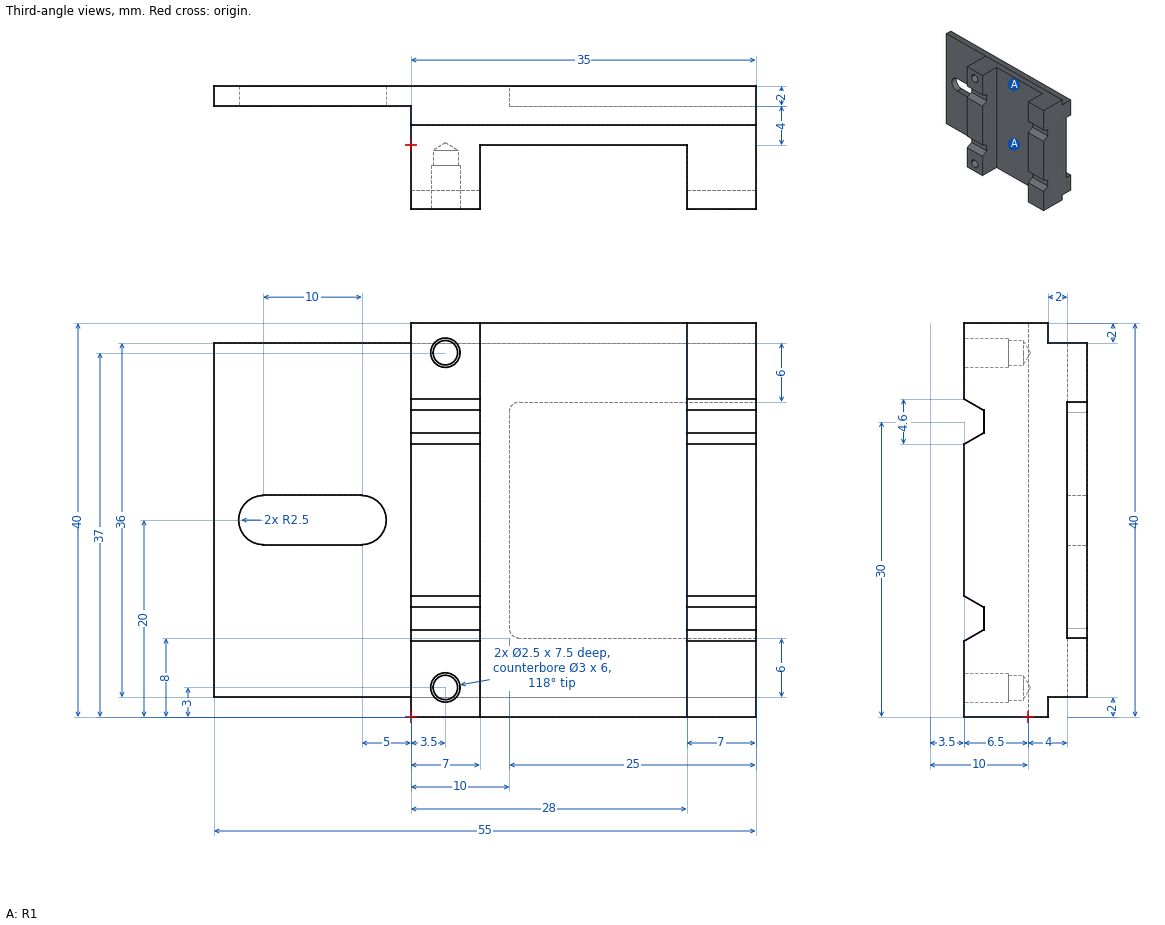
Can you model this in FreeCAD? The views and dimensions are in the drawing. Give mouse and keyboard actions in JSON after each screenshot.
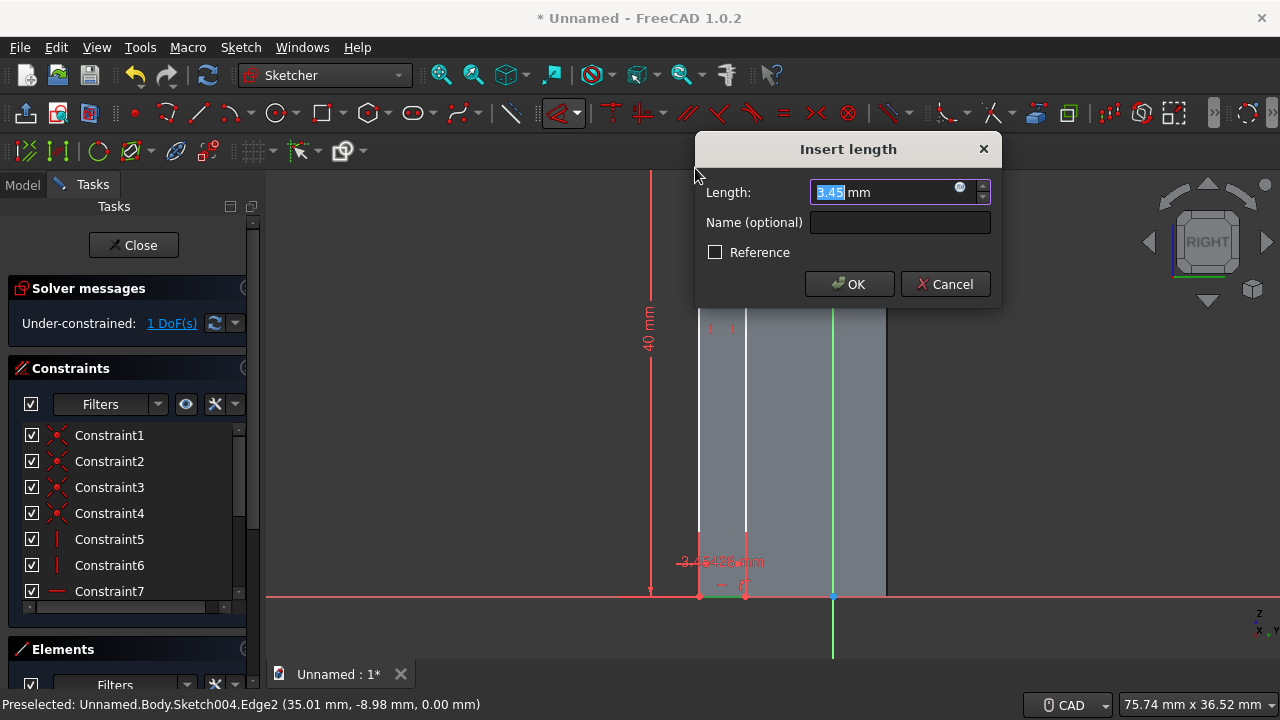
{"action": "type", "text": "3.5"}
{"action": "key", "text": "Return"}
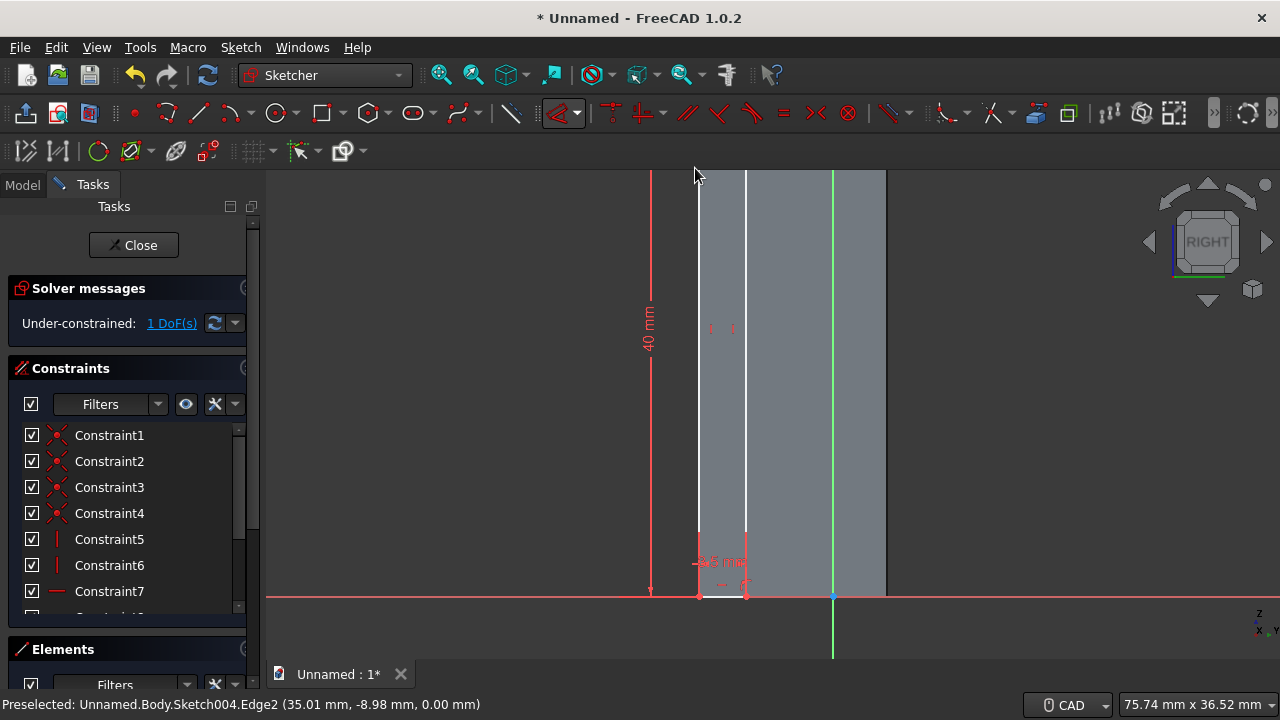
{"action": "scroll", "coordinate": [629, 519], "scroll_direction": "down", "scroll_amount": 3}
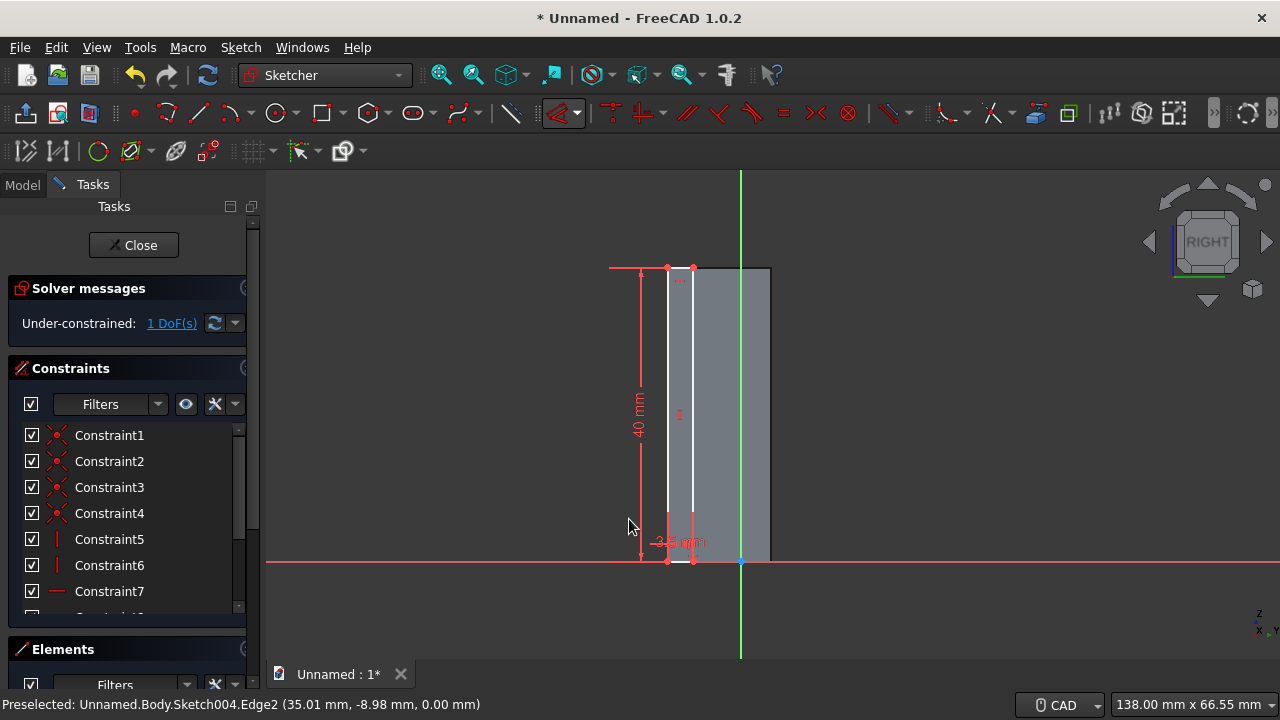
{"action": "left_click", "coordinate": [668, 268]}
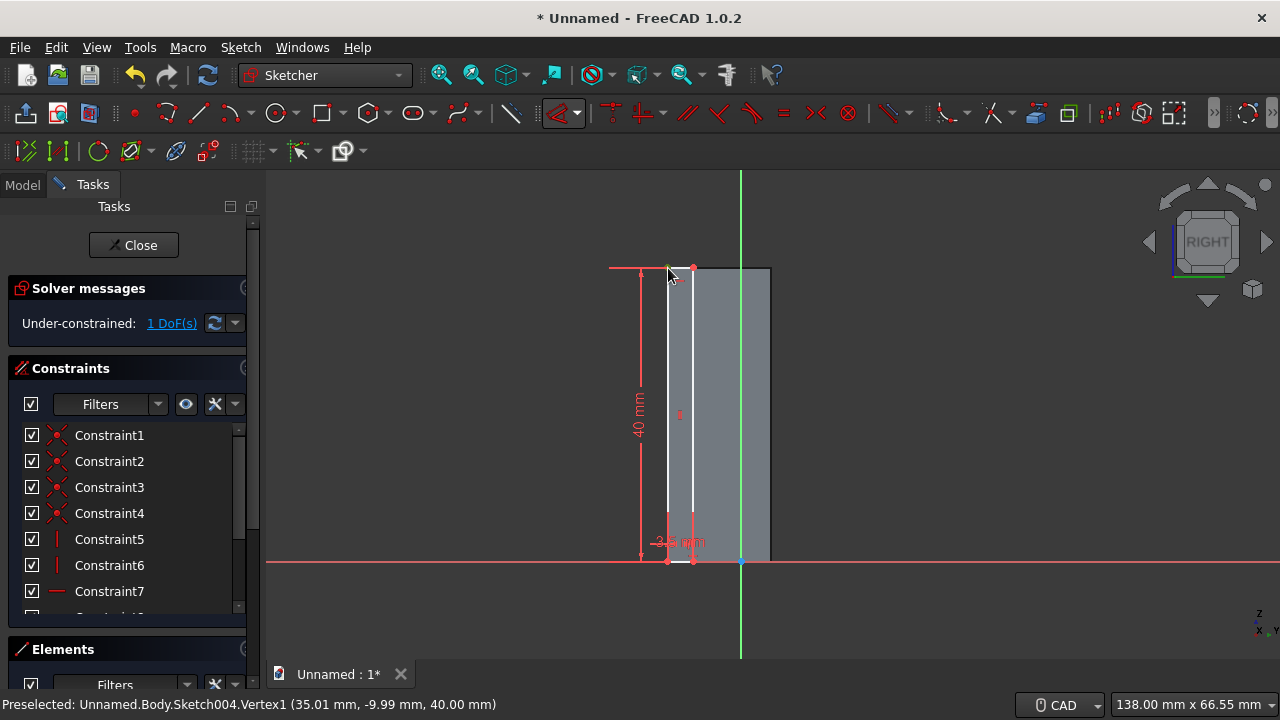
{"action": "left_click", "coordinate": [580, 114]}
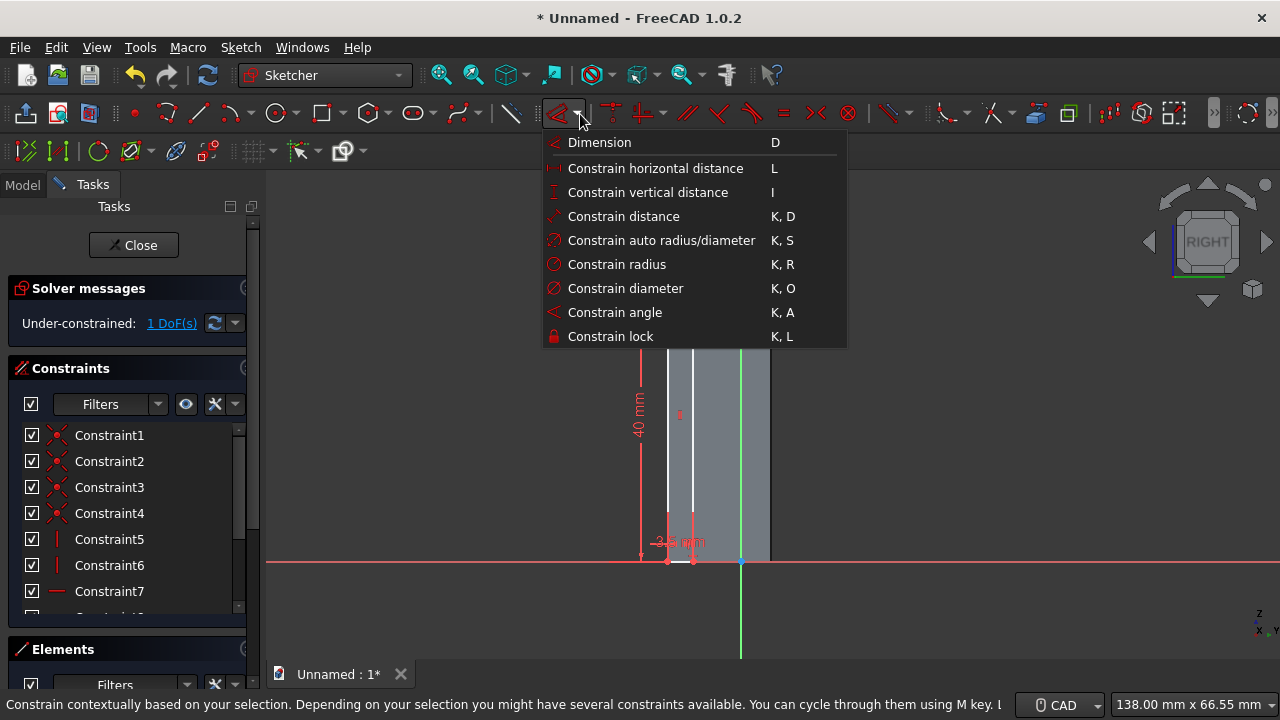
{"action": "left_click", "coordinate": [695, 168]}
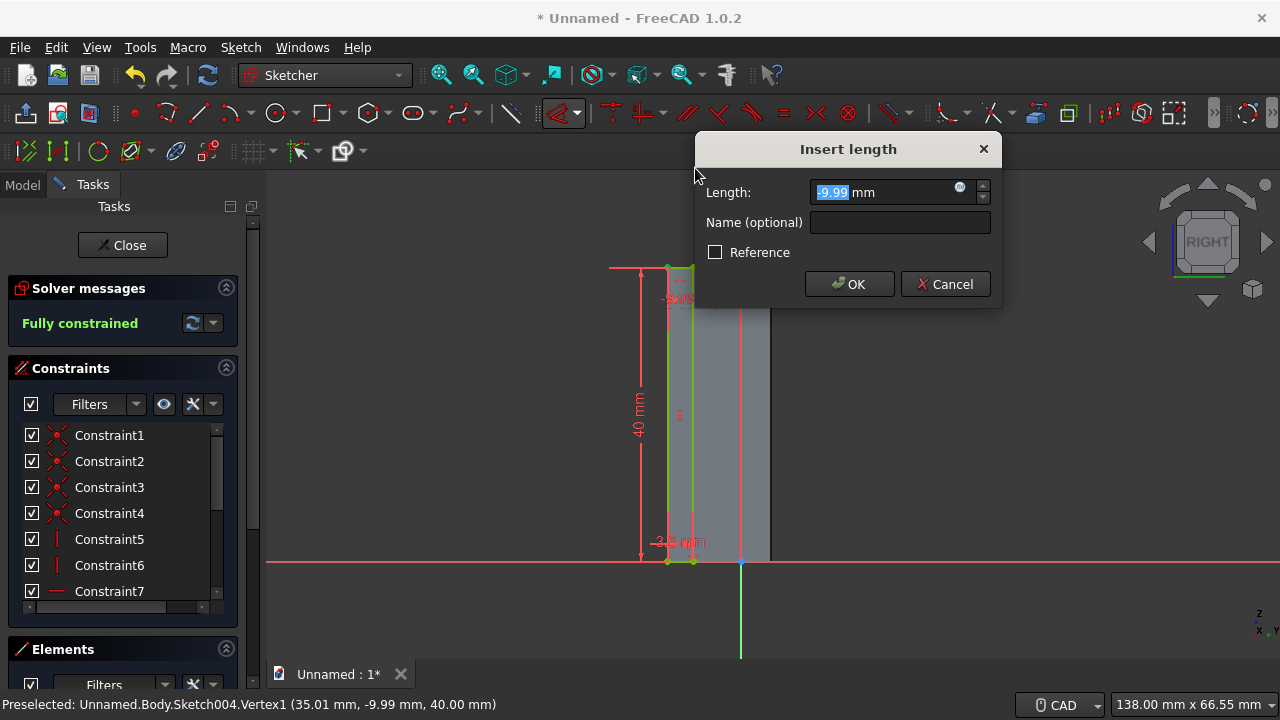
{"action": "type", "text": "-10"}
{"action": "key", "text": "Return"}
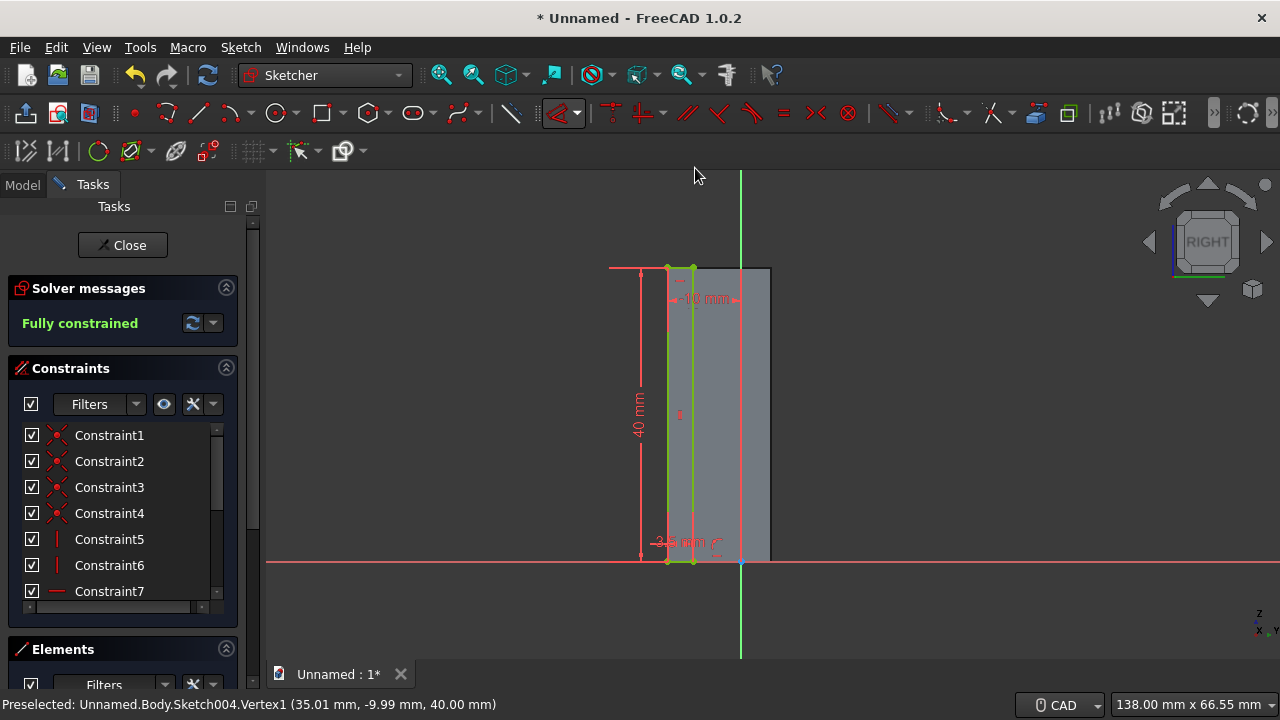
{"action": "left_click", "coordinate": [123, 245]}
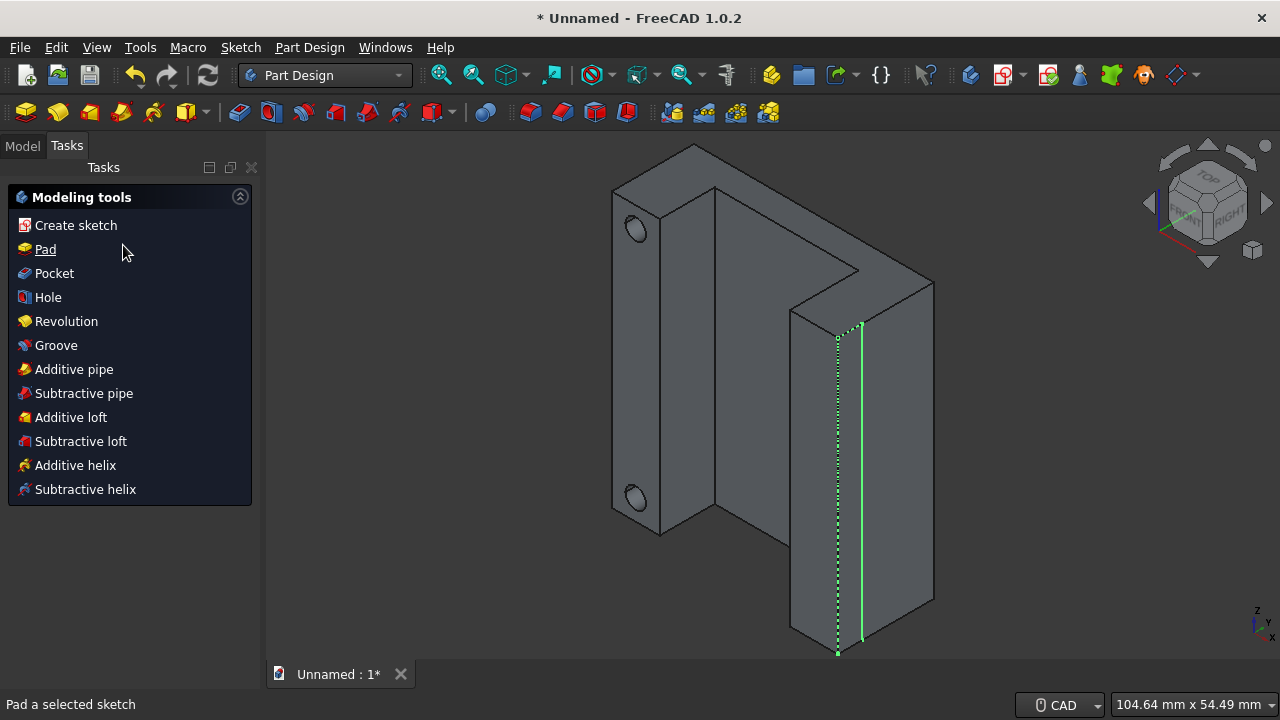
{"action": "left_click", "coordinate": [240, 112]}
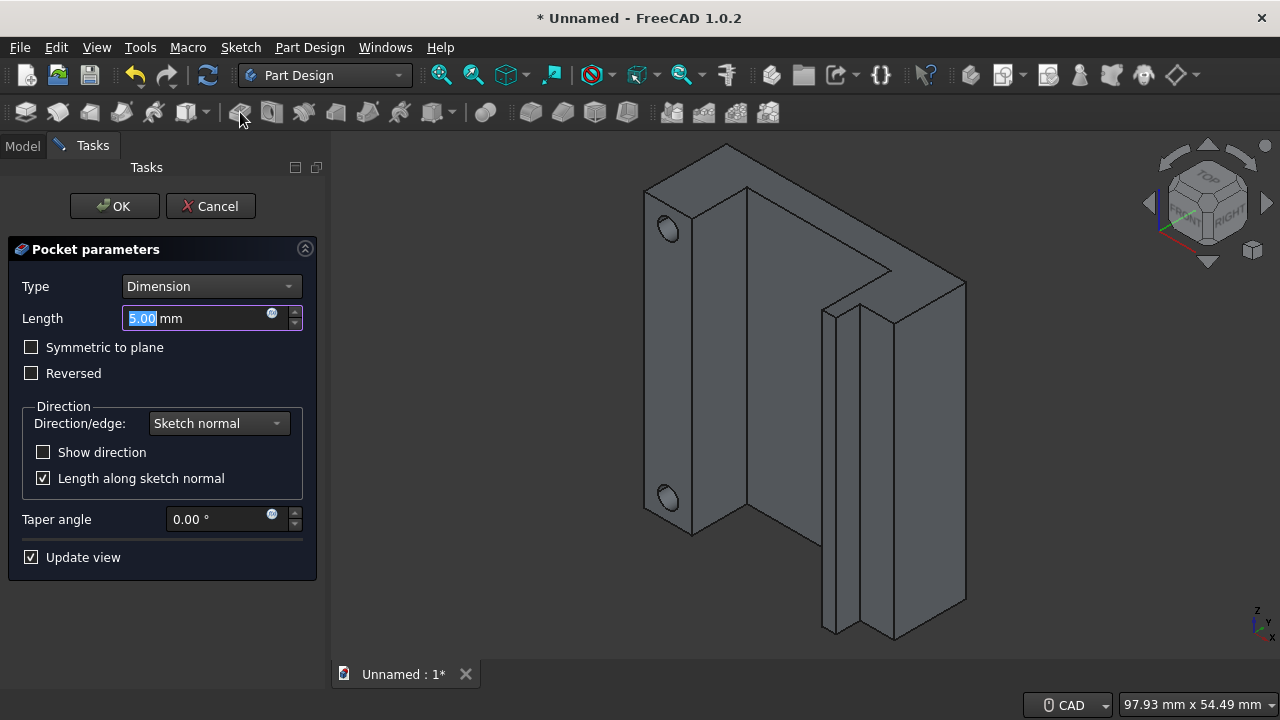
{"action": "left_click", "coordinate": [212, 286]}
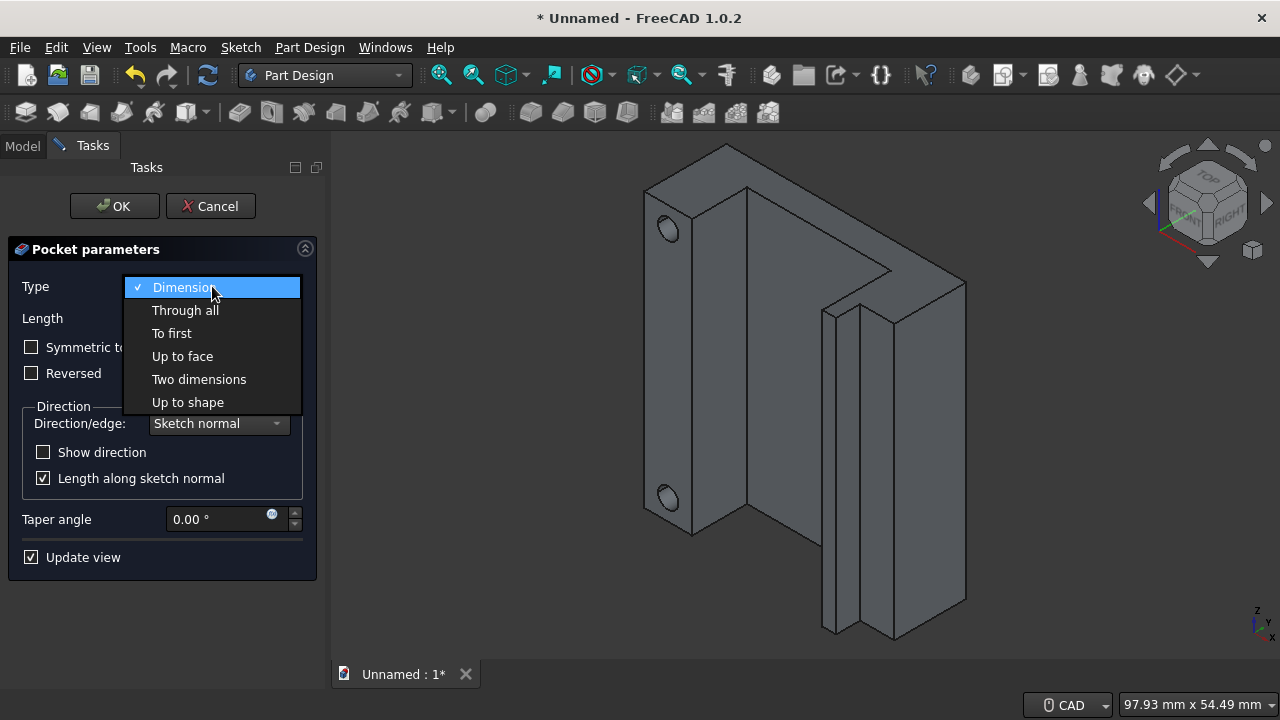
{"action": "left_click", "coordinate": [212, 310]}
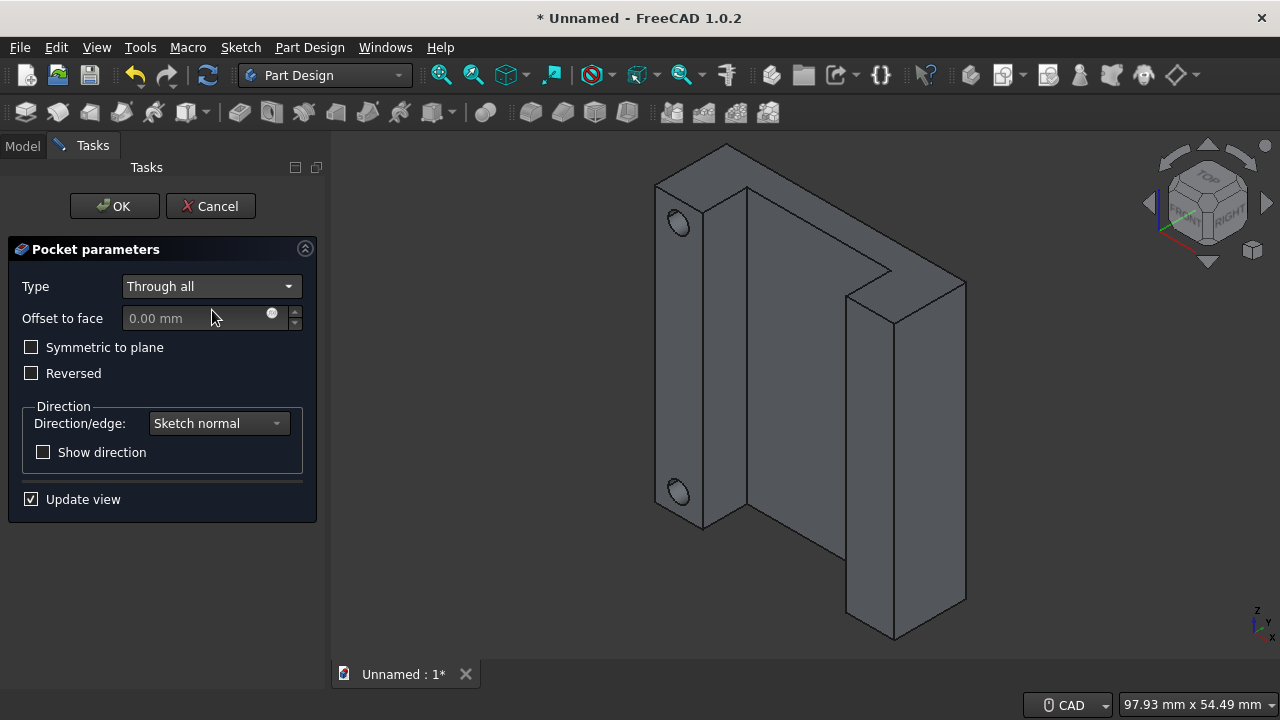
{"action": "left_click", "coordinate": [115, 206]}